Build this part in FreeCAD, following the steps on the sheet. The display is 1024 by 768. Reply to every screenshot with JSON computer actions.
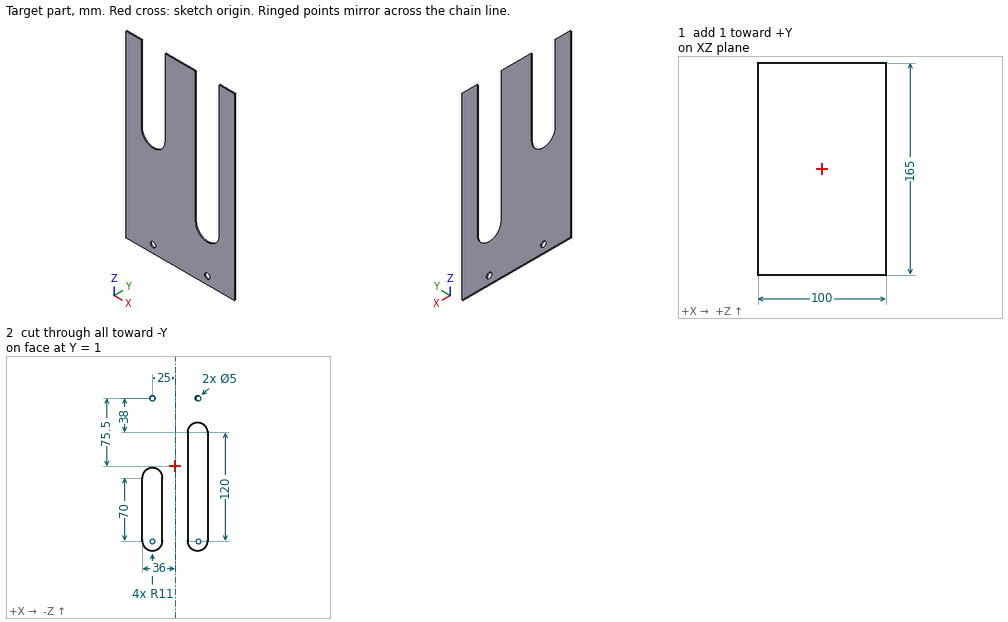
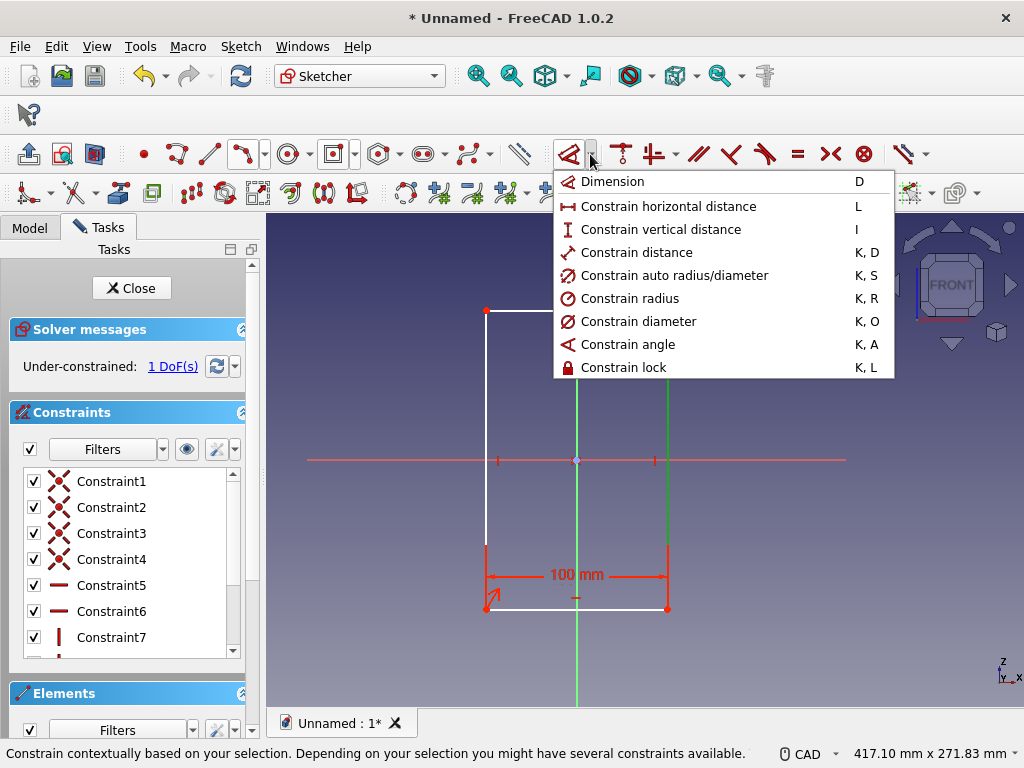
{"action": "left_click", "coordinate": [724, 230]}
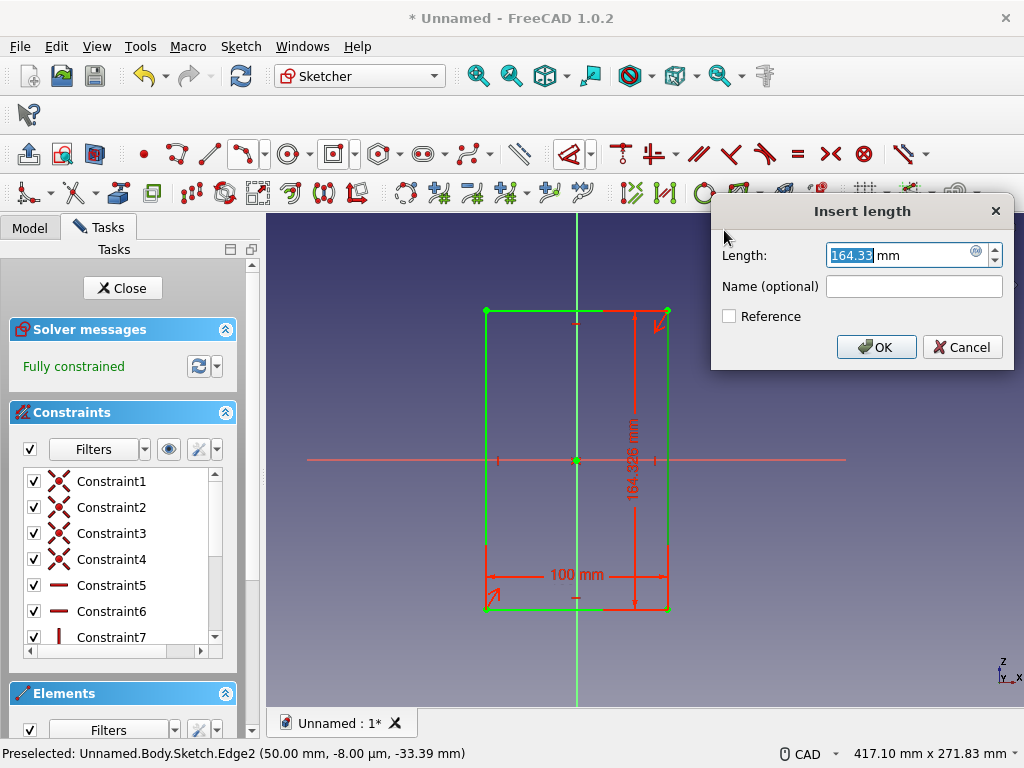
{"action": "type", "text": "165"}
{"action": "key", "text": "Return"}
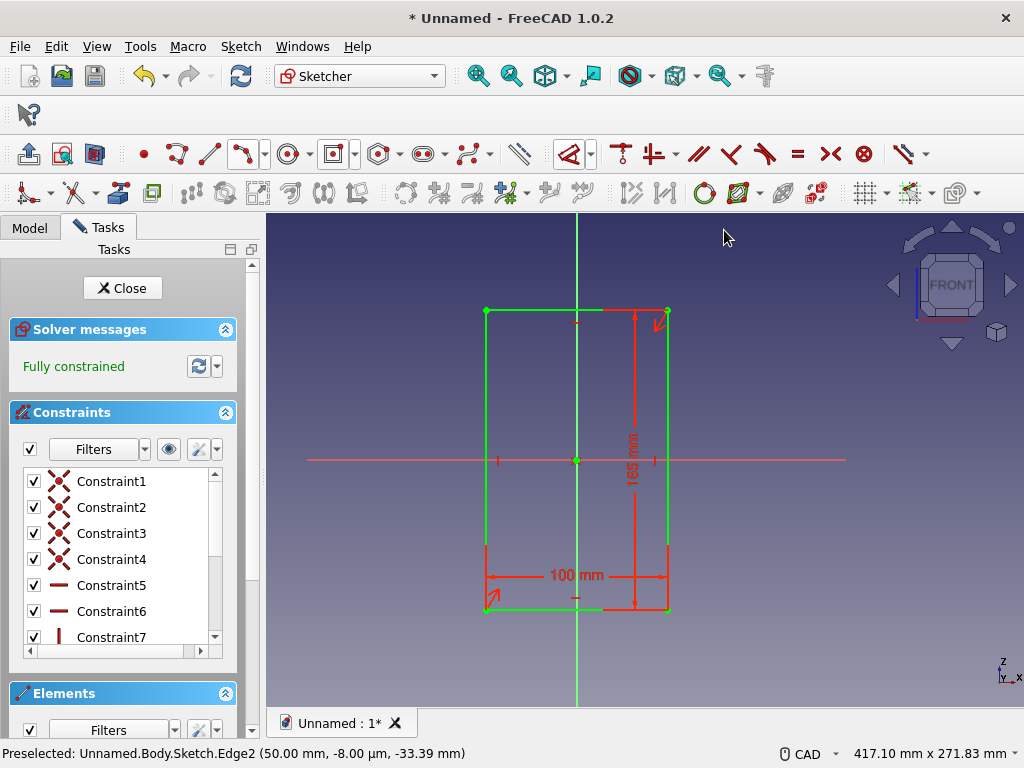
{"action": "left_click", "coordinate": [123, 288]}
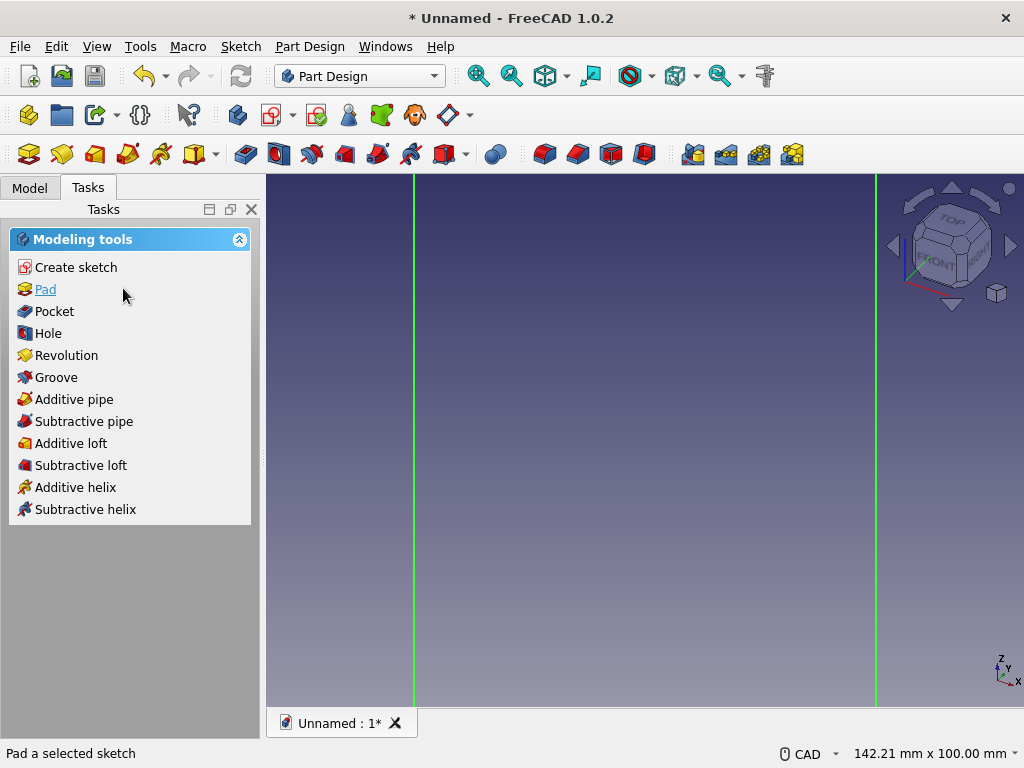
{"action": "left_click", "coordinate": [29, 154]}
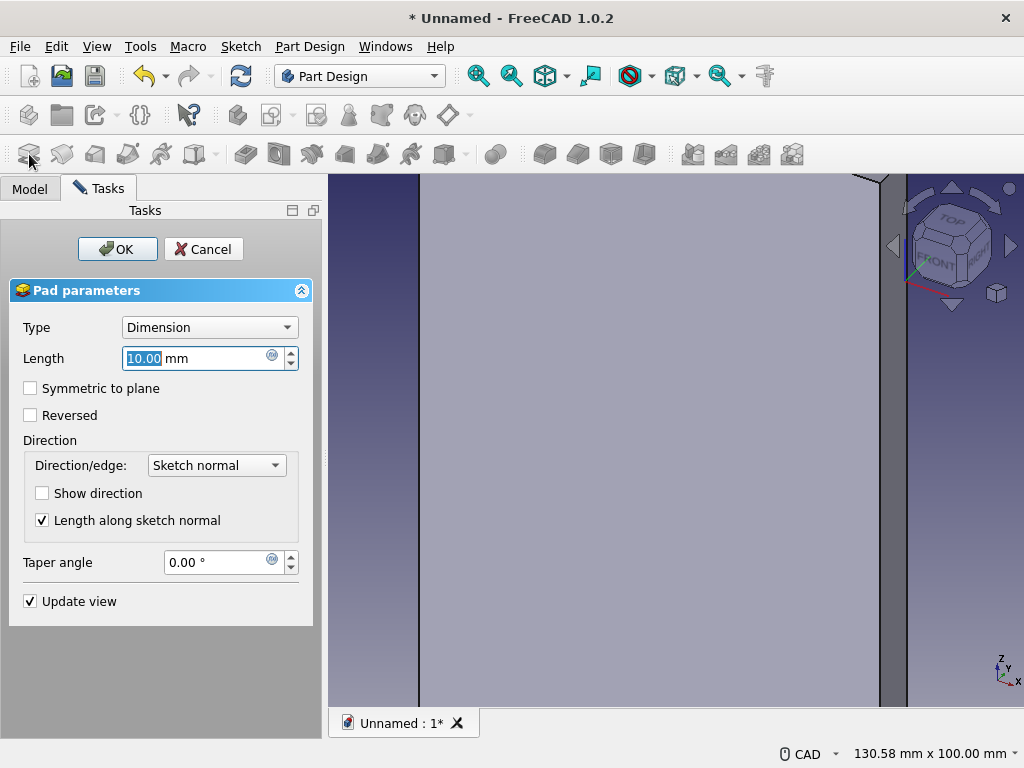
{"action": "type", "text": "1"}
{"action": "key", "text": "Tab"}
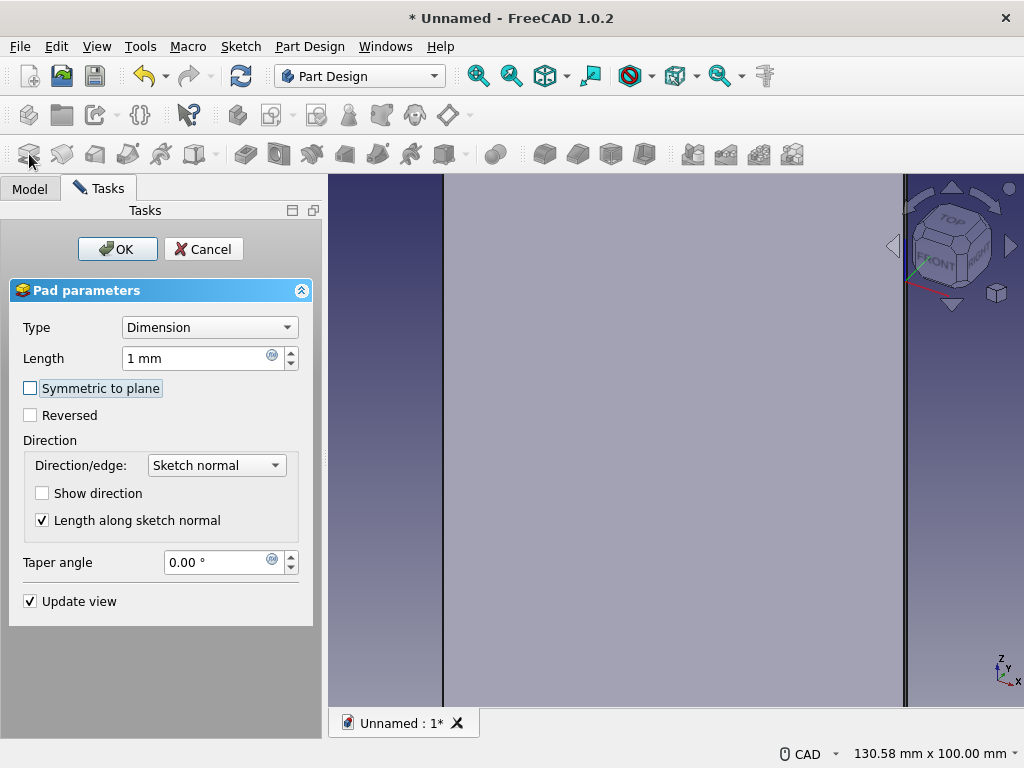
{"action": "left_click", "coordinate": [31, 415]}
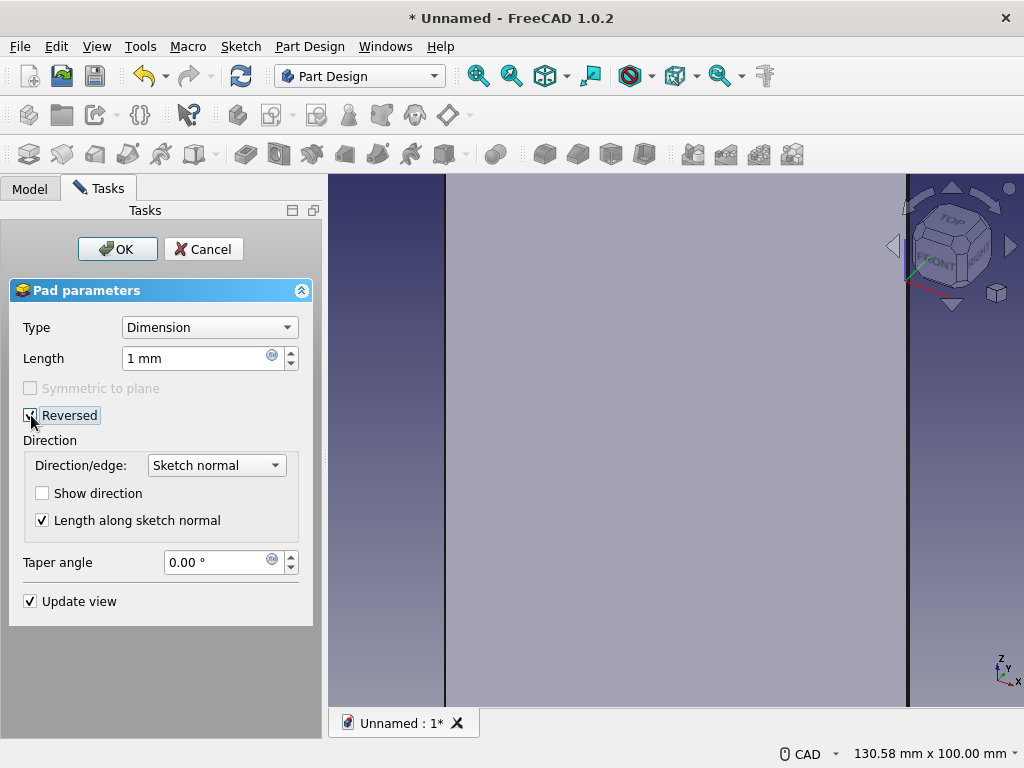
{"action": "left_click", "coordinate": [118, 249]}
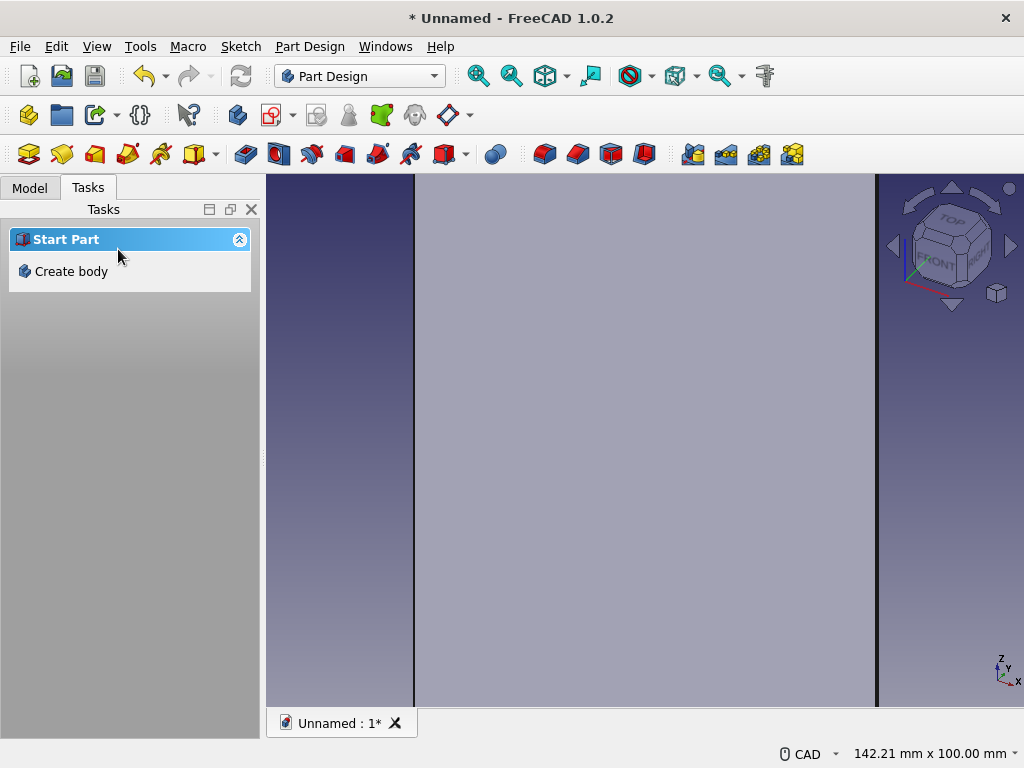
{"action": "left_click", "coordinate": [479, 76]}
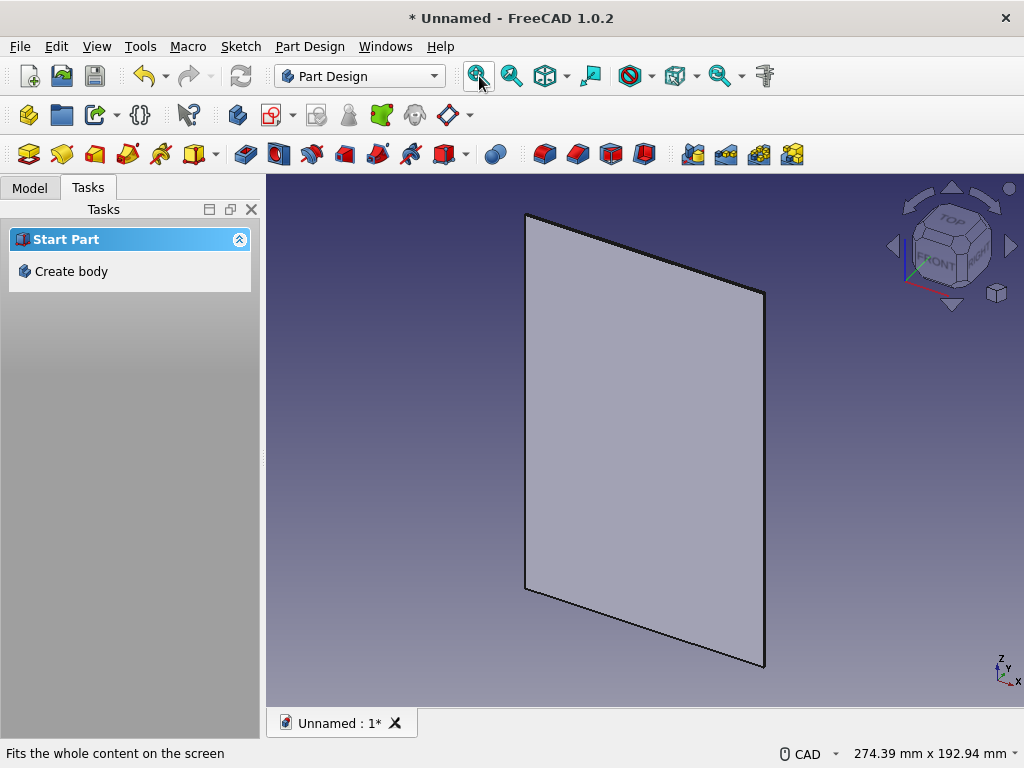
{"action": "key", "text": "4"}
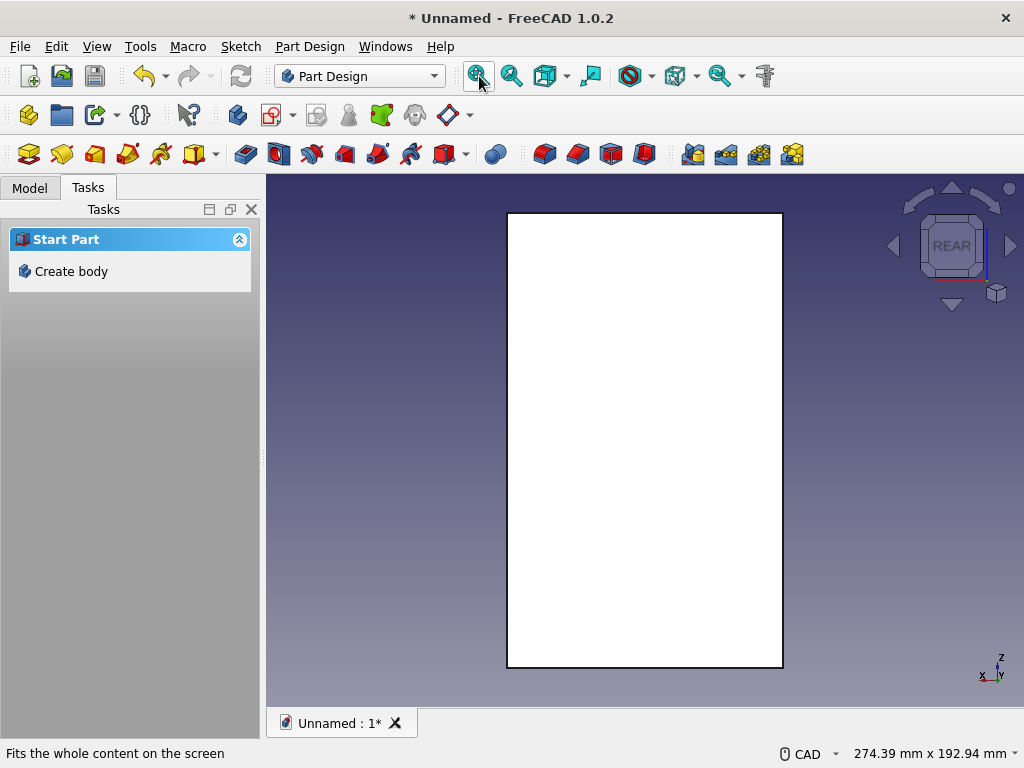
{"action": "left_click", "coordinate": [645, 374]}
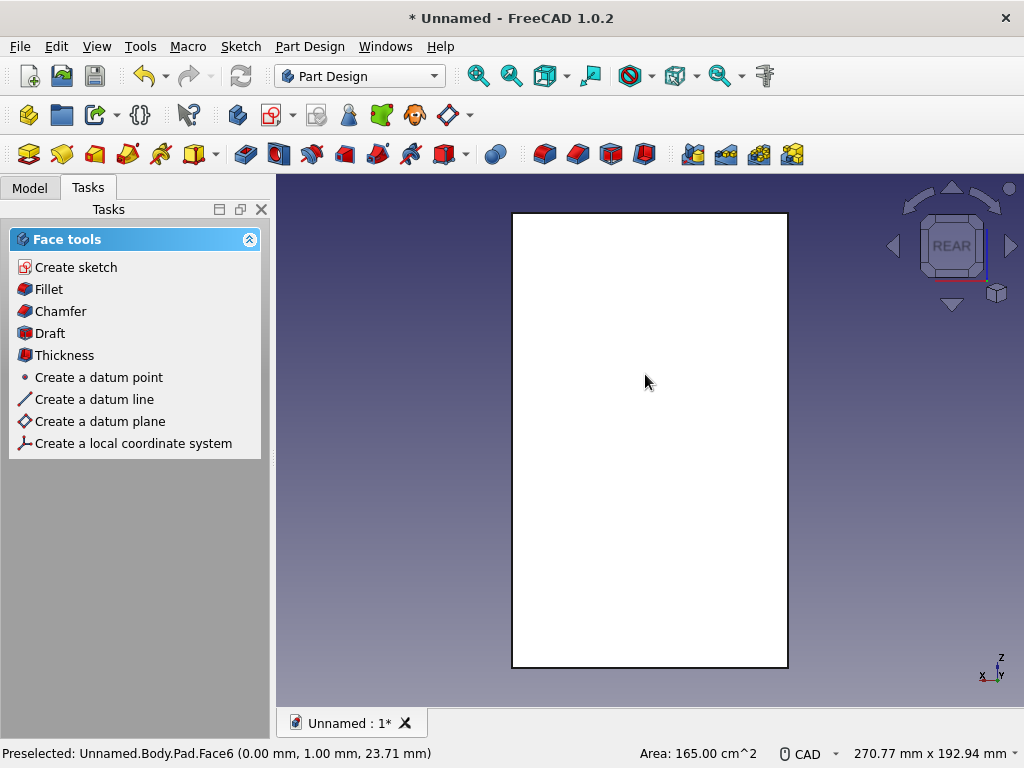
{"action": "left_click", "coordinate": [270, 116]}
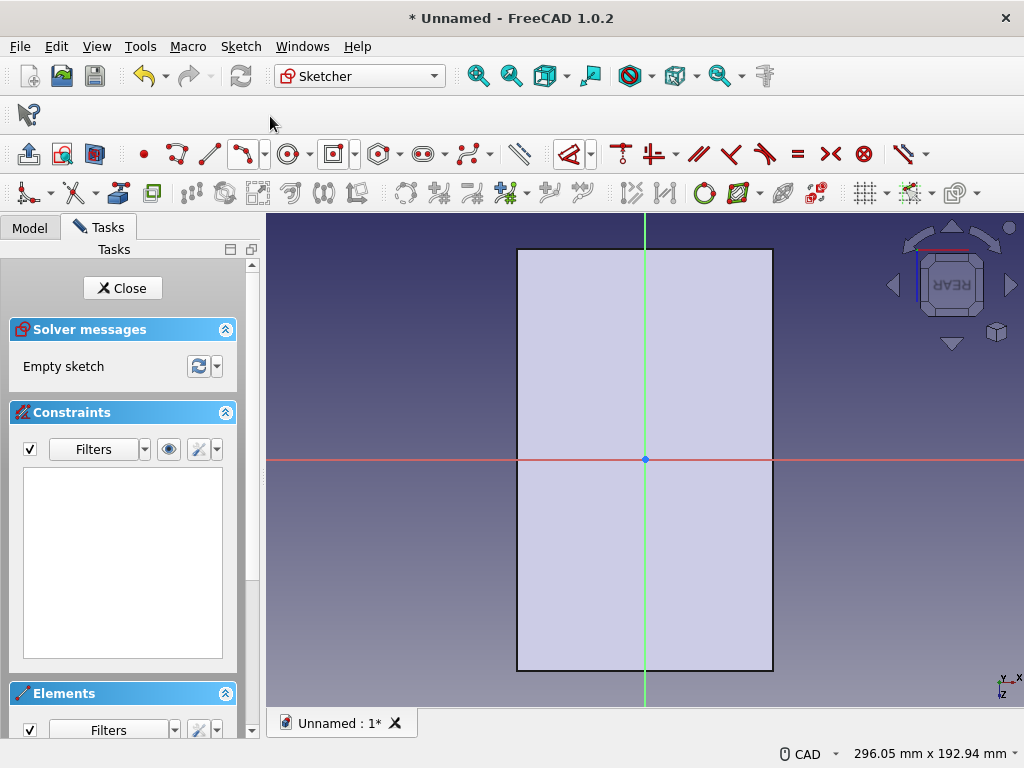
{"action": "scroll", "coordinate": [437, 420], "scroll_direction": "down", "scroll_amount": 2}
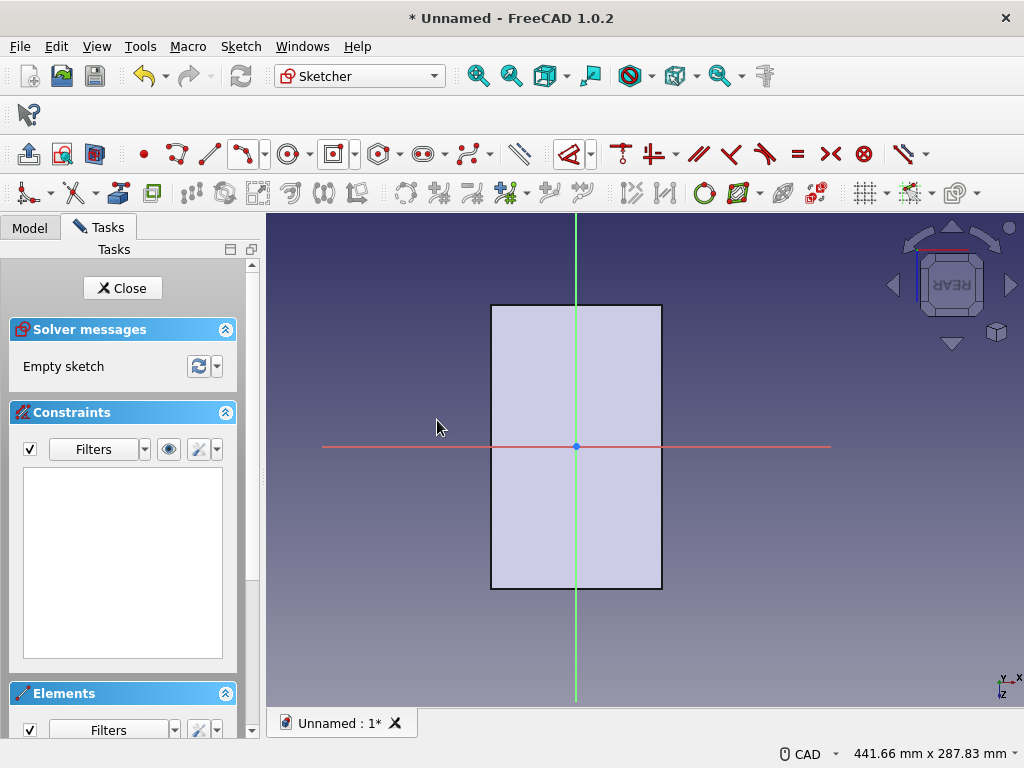
{"action": "left_click", "coordinate": [422, 154]}